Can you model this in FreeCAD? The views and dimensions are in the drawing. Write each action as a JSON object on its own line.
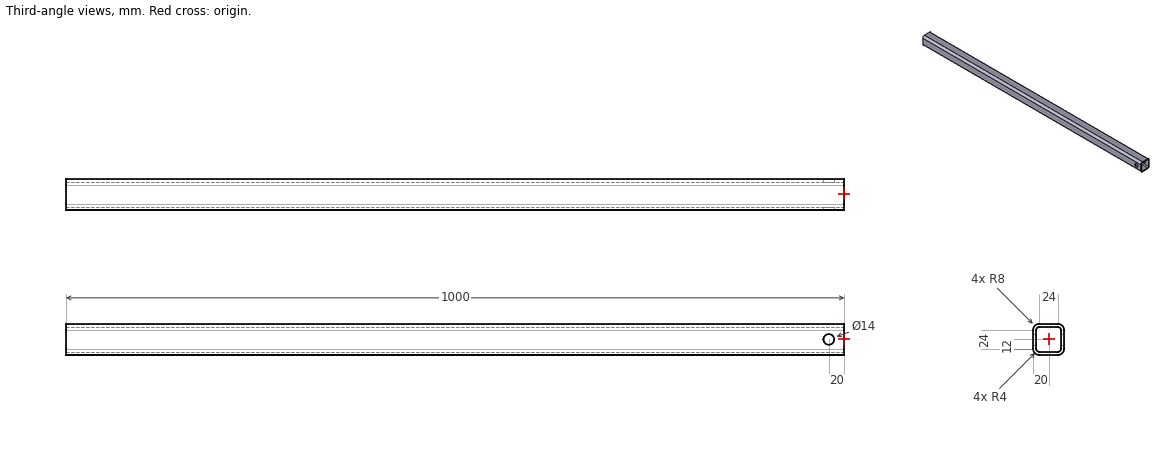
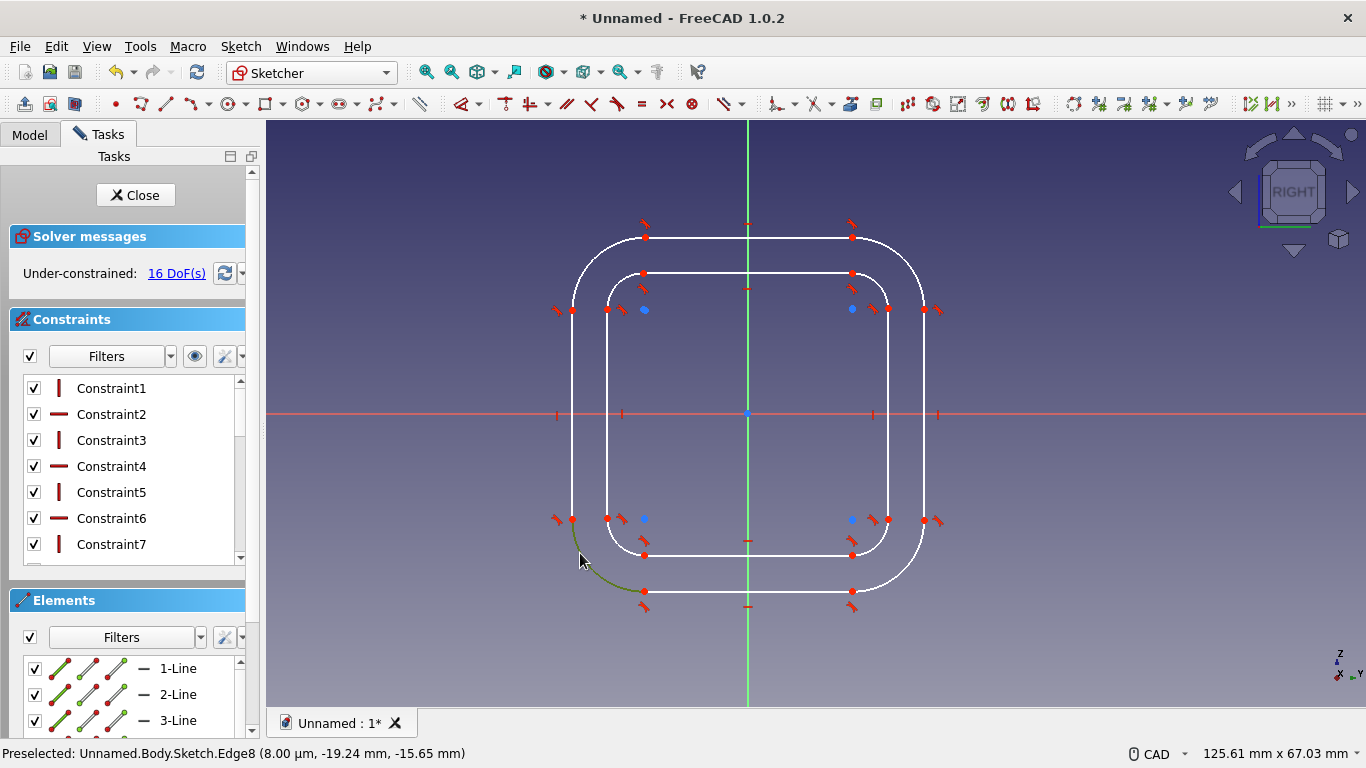
{"action": "left_click", "coordinate": [612, 535]}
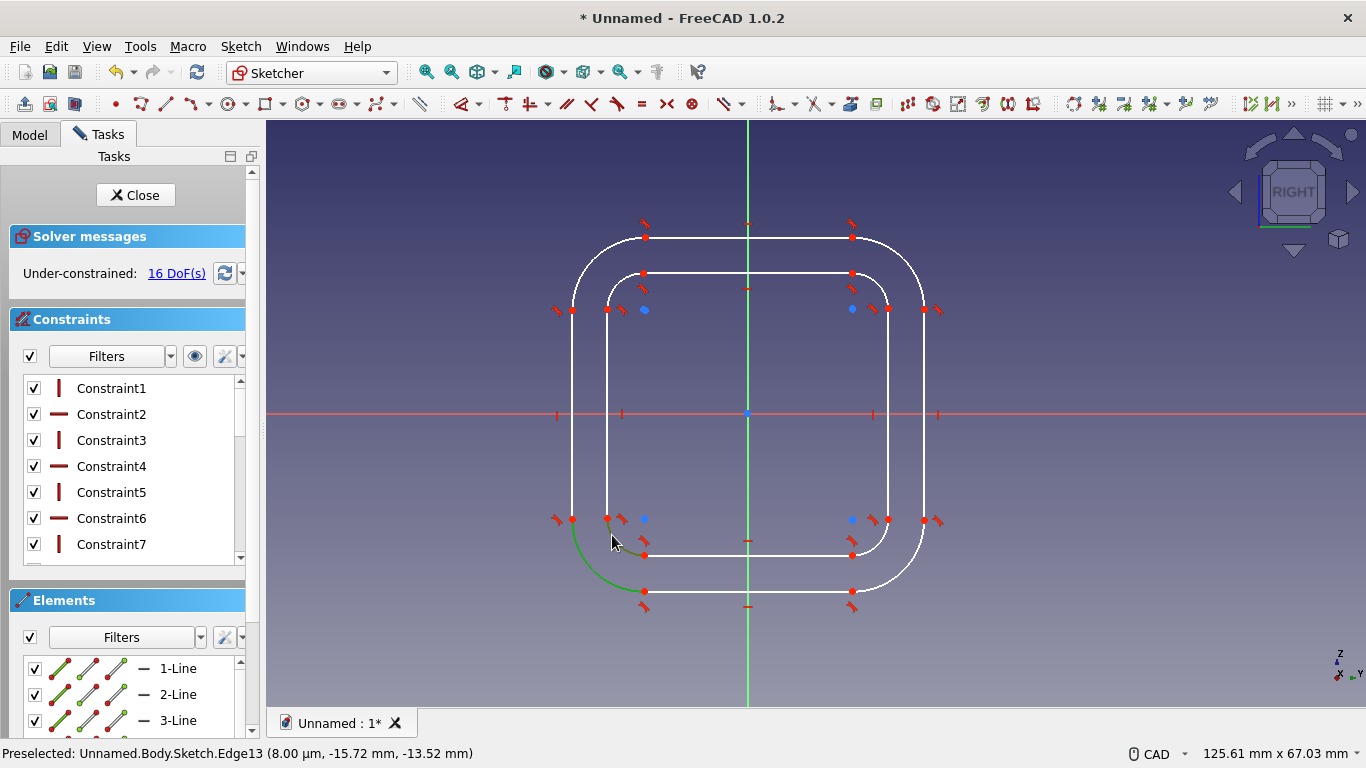
{"action": "key", "text": "c"}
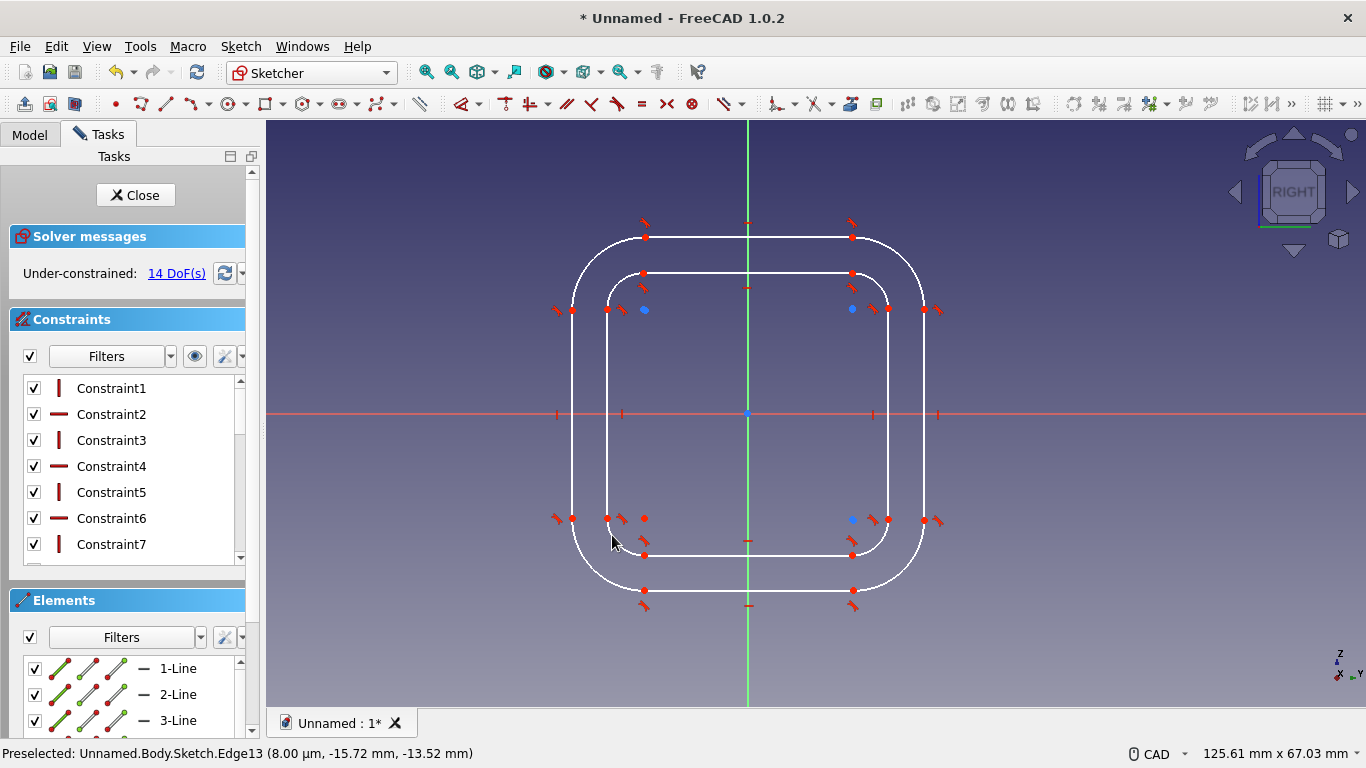
{"action": "left_click", "coordinate": [885, 583]}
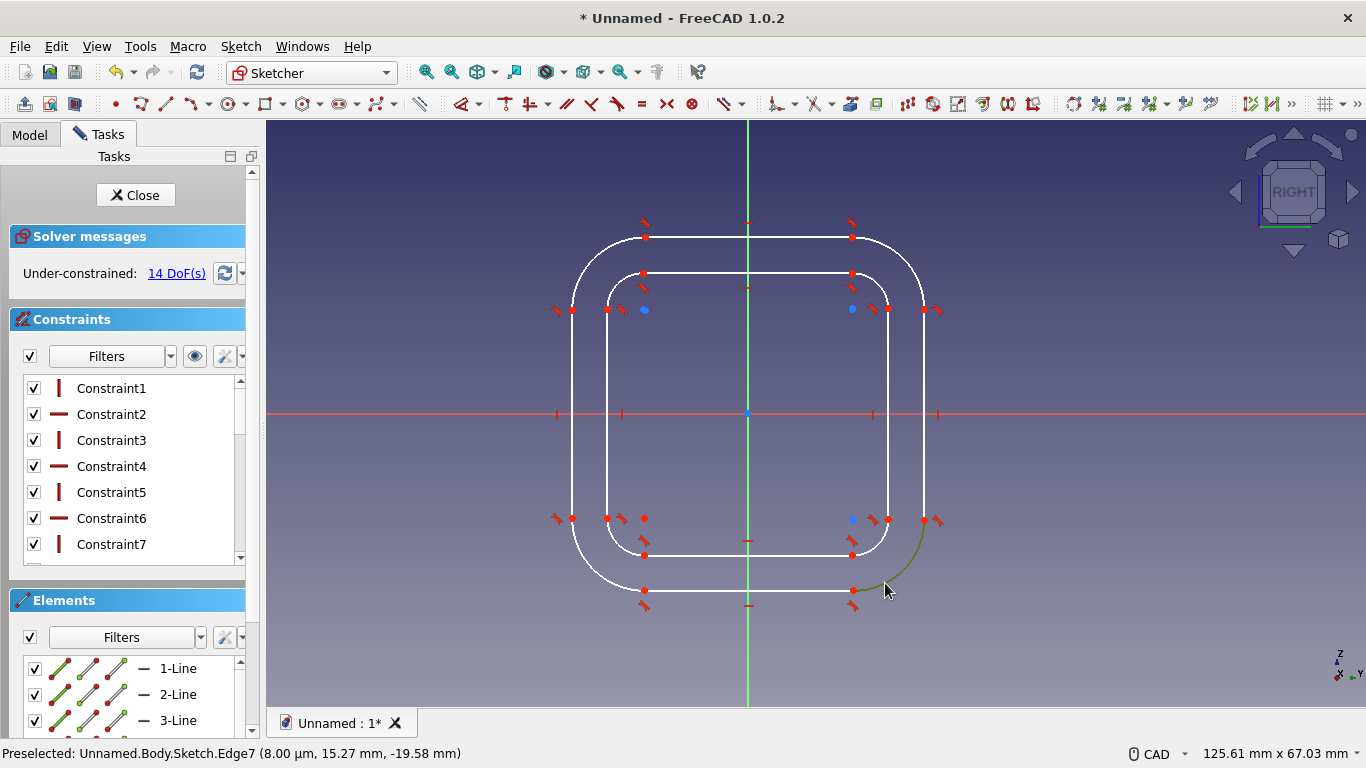
{"action": "left_click", "coordinate": [869, 552]}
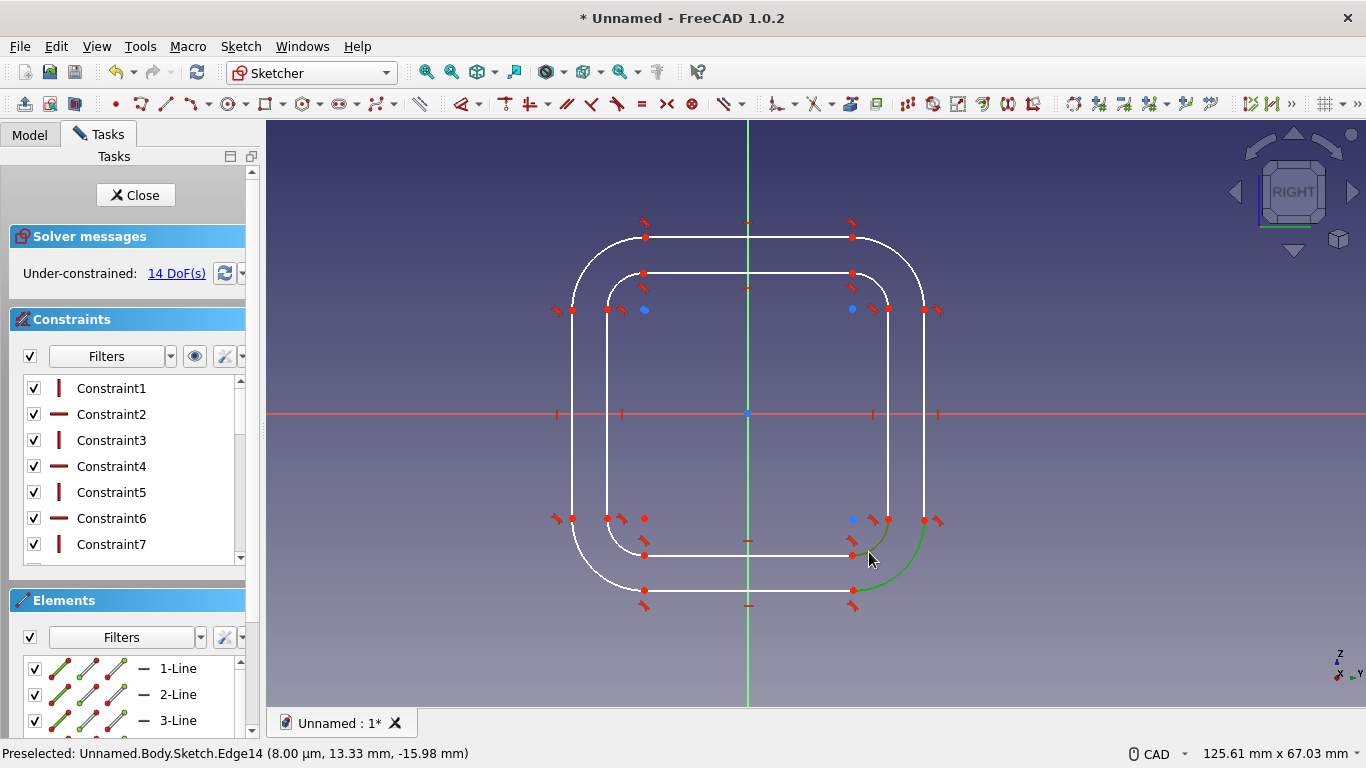
{"action": "left_click", "coordinate": [505, 104]}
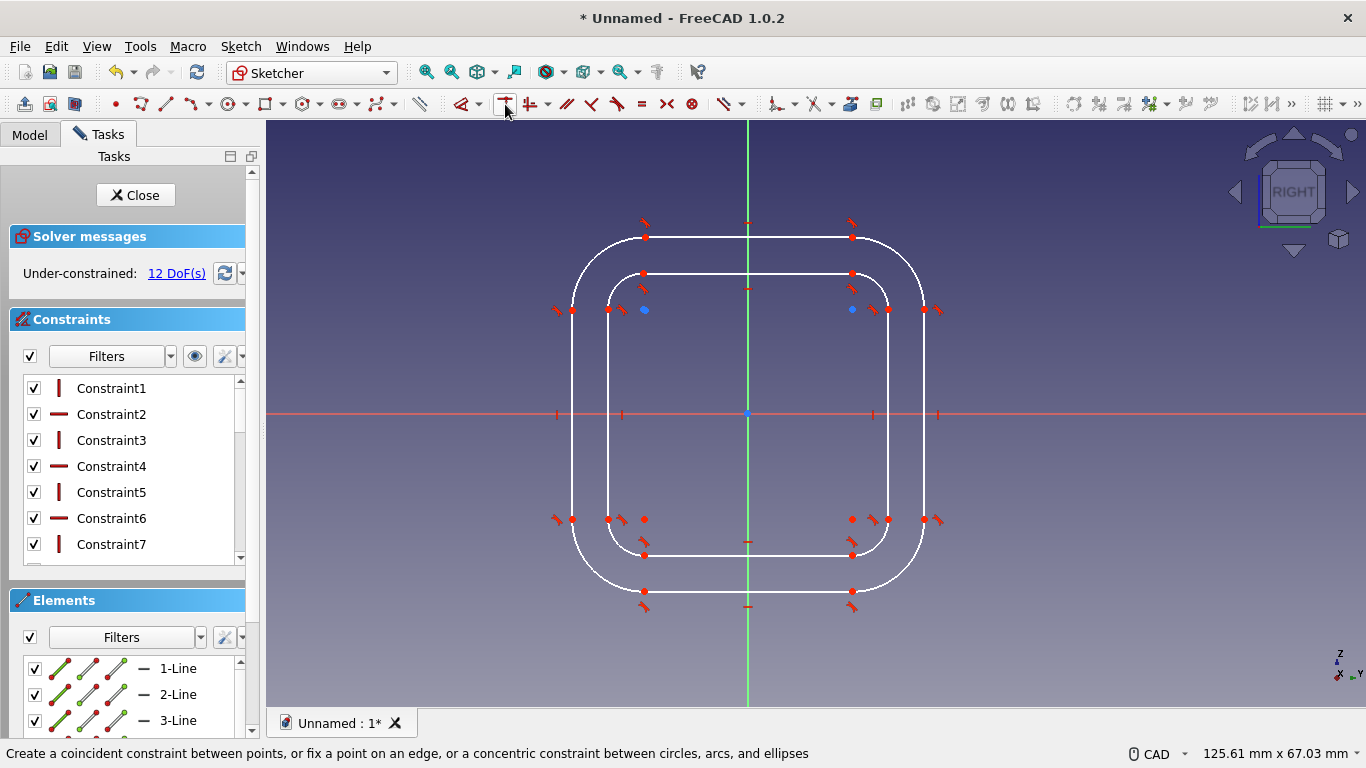
{"action": "left_click", "coordinate": [916, 277]}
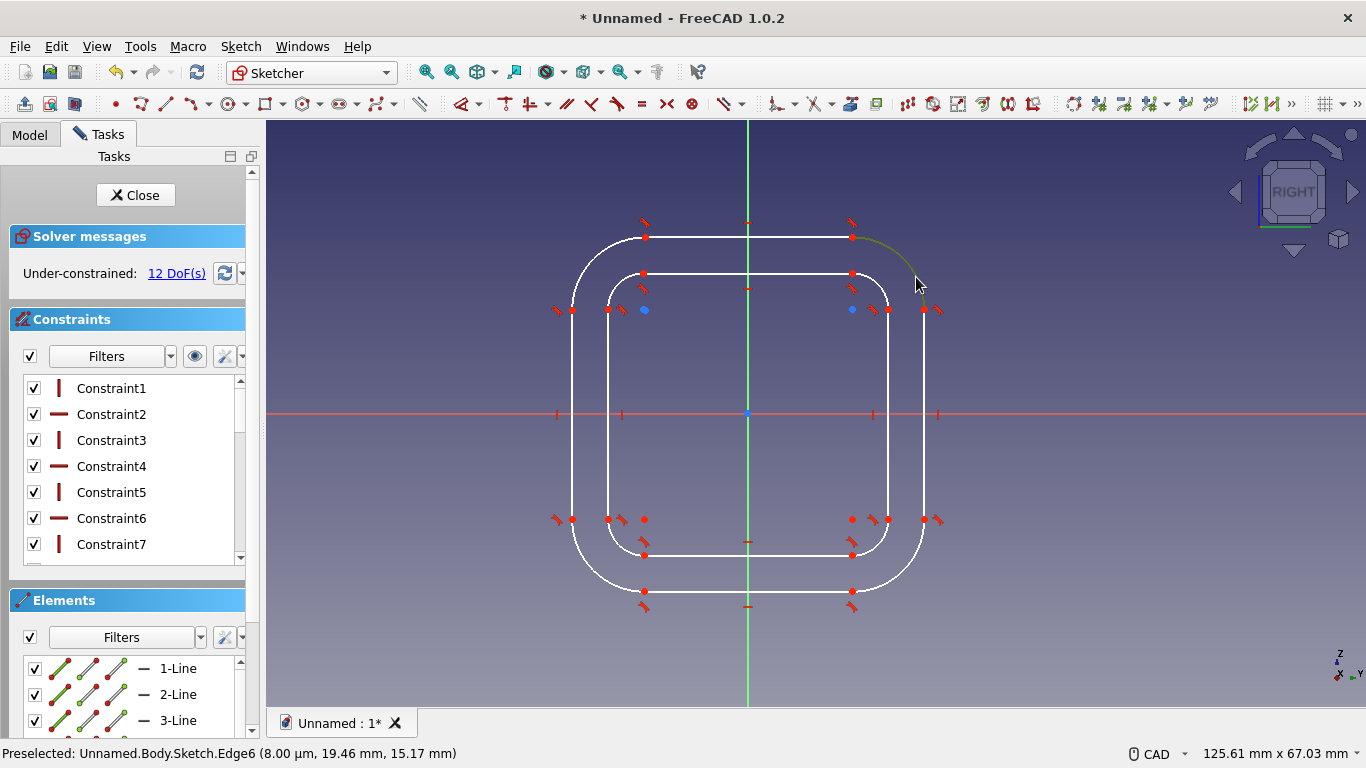
{"action": "left_click", "coordinate": [884, 293]}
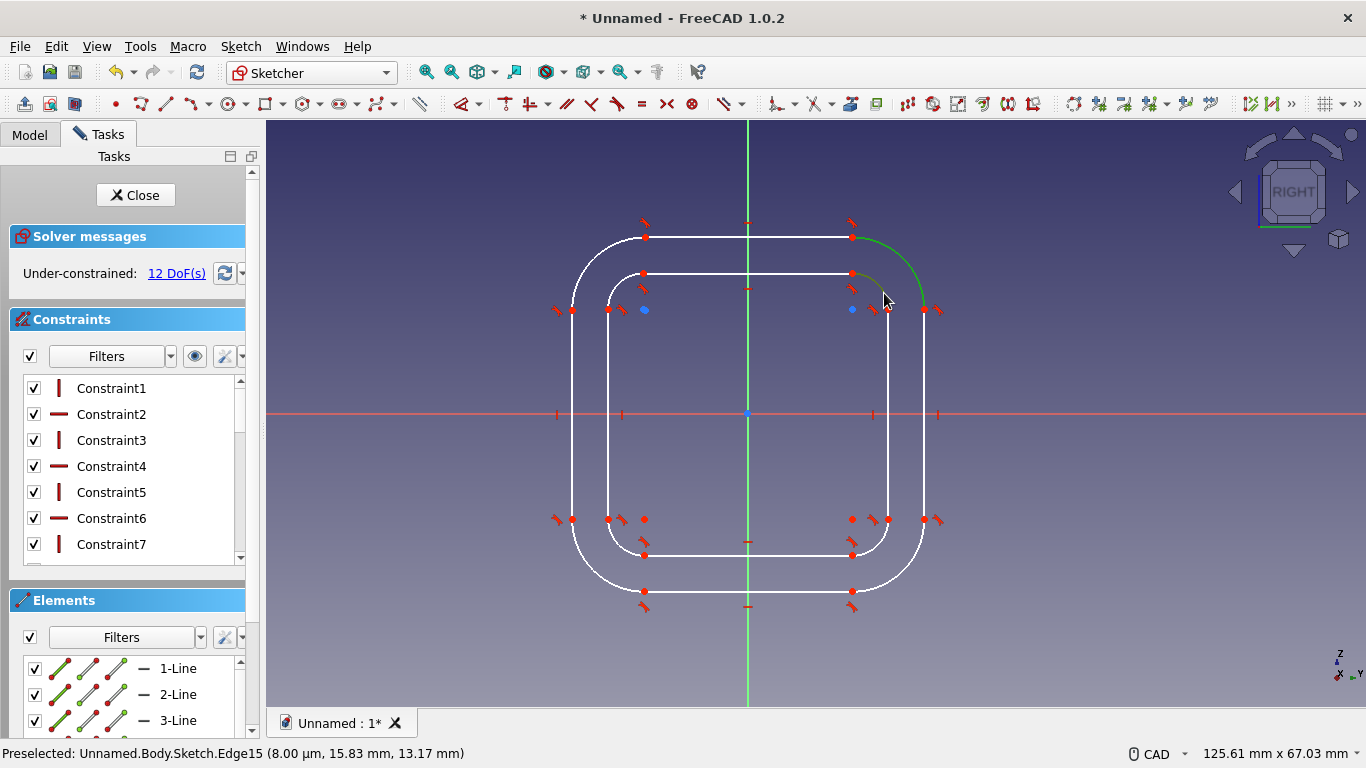
{"action": "key", "text": "c"}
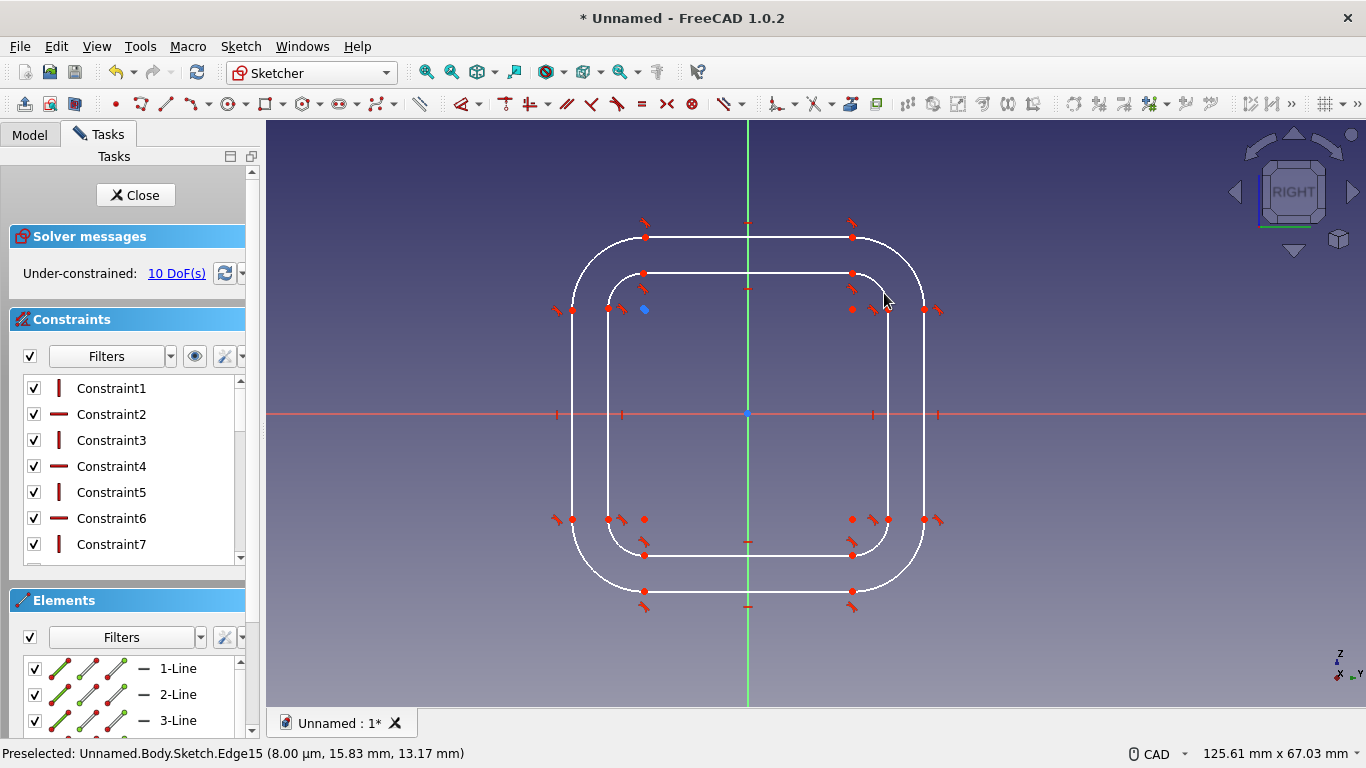
{"action": "left_click", "coordinate": [612, 245]}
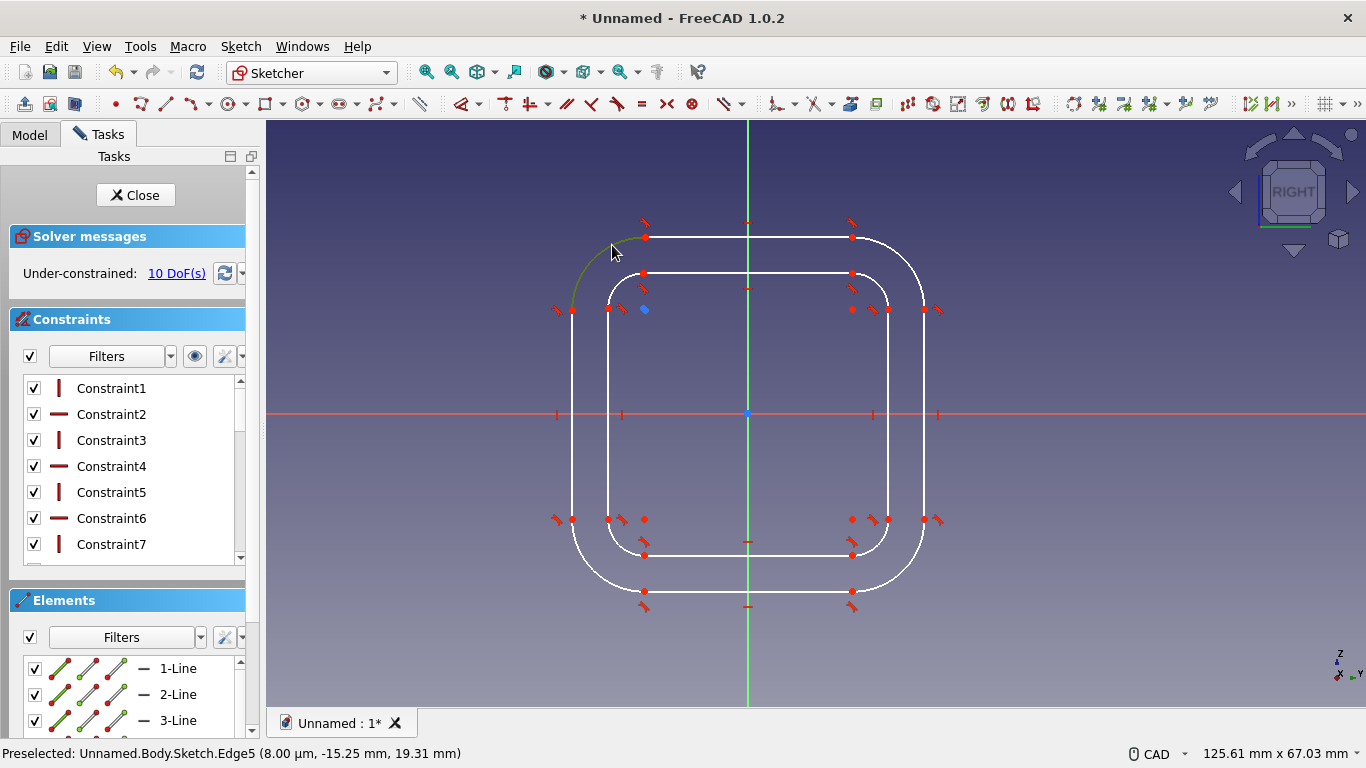
{"action": "left_click", "coordinate": [916, 277]}